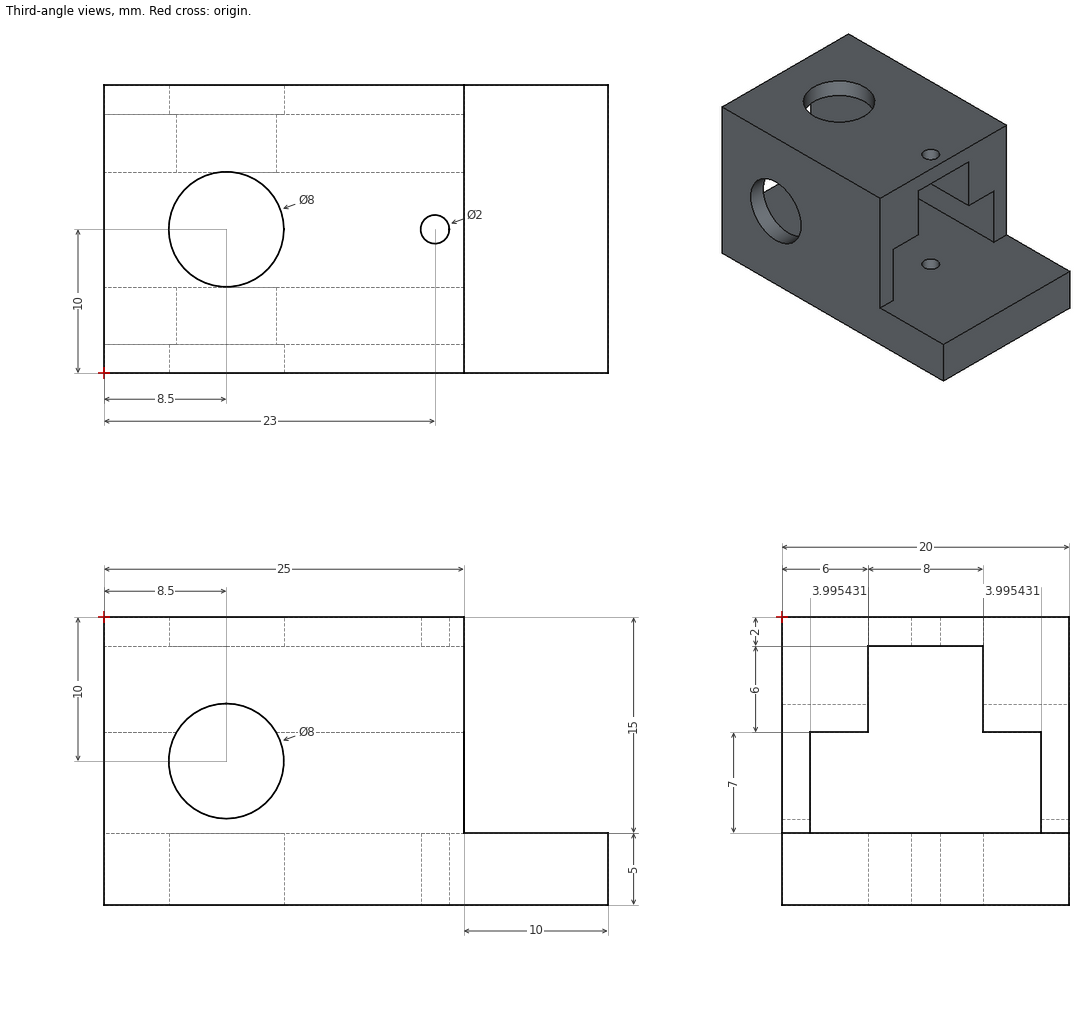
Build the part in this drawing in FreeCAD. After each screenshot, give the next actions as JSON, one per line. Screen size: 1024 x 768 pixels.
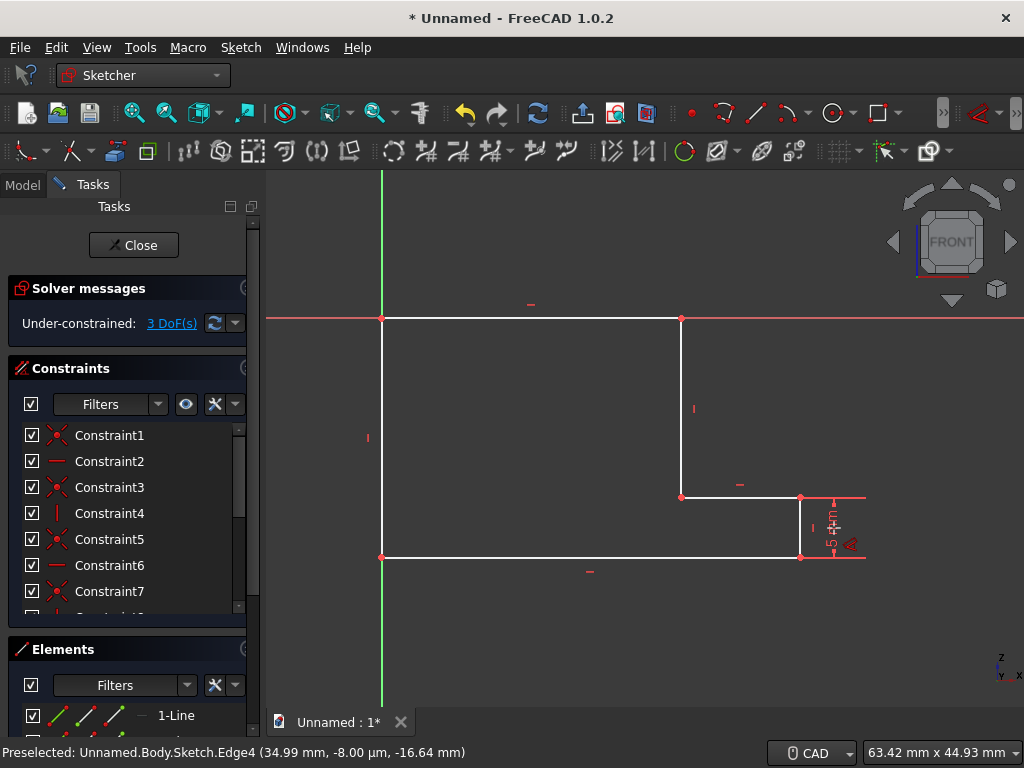
{"action": "left_click", "coordinate": [472, 318]}
{"action": "left_click", "coordinate": [531, 284]}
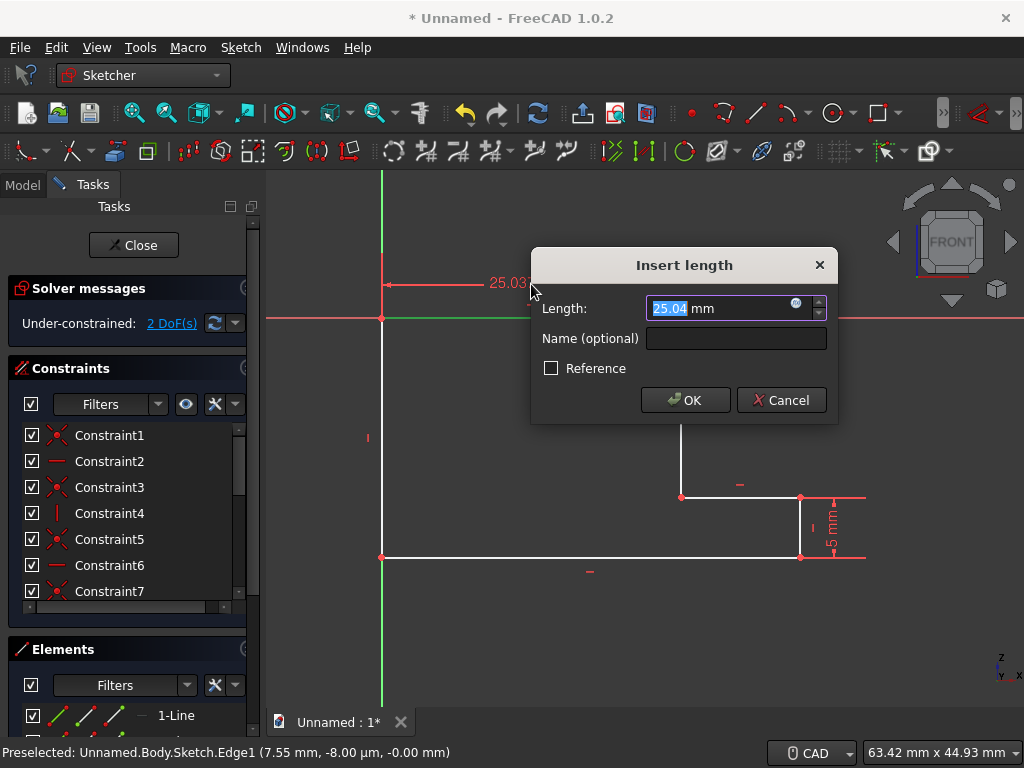
{"action": "type", "text": "25"}
{"action": "key", "text": "Return"}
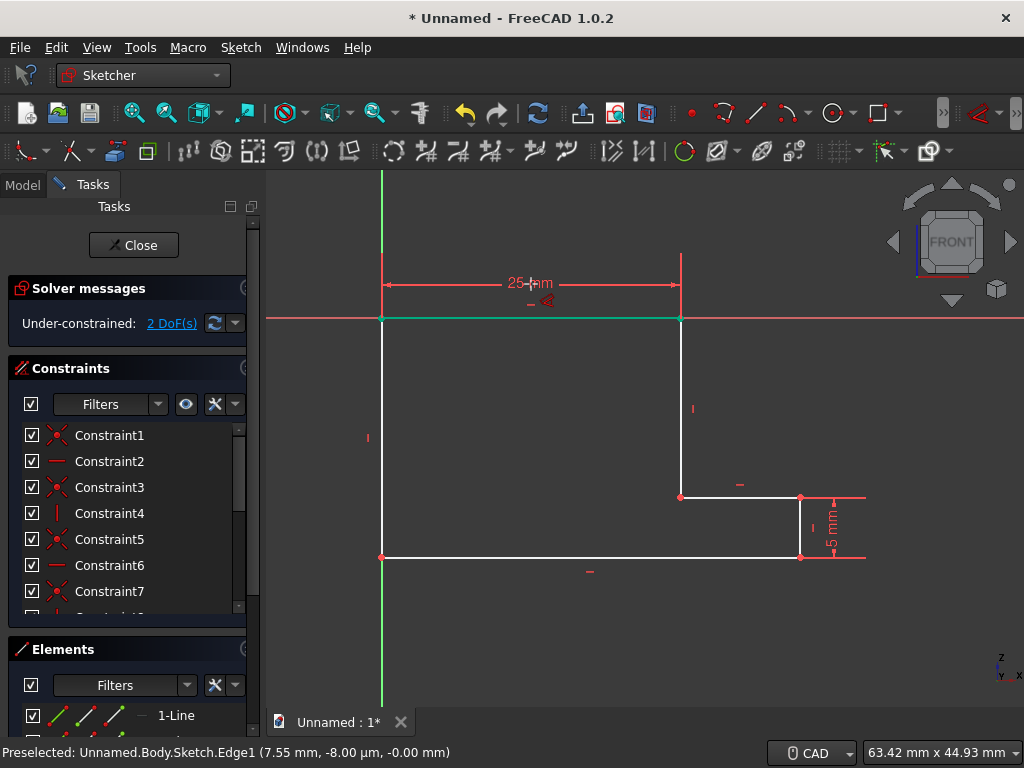
{"action": "left_click", "coordinate": [681, 372]}
{"action": "left_click", "coordinate": [715, 408]}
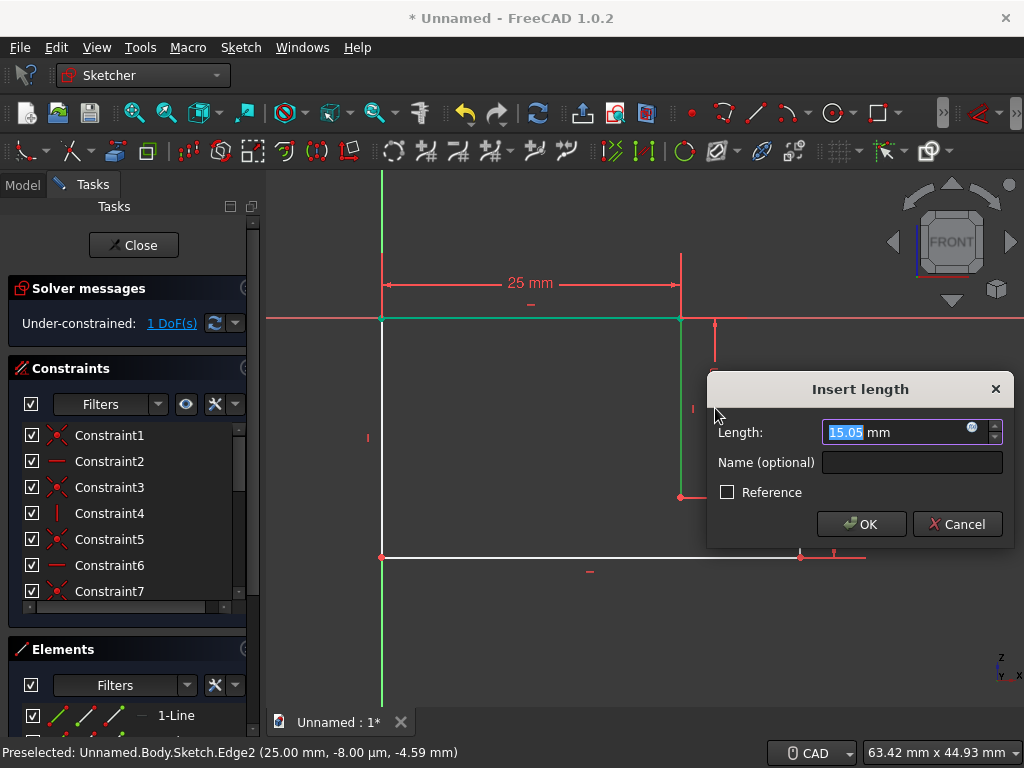
{"action": "type", "text": "15"}
{"action": "key", "text": "Return"}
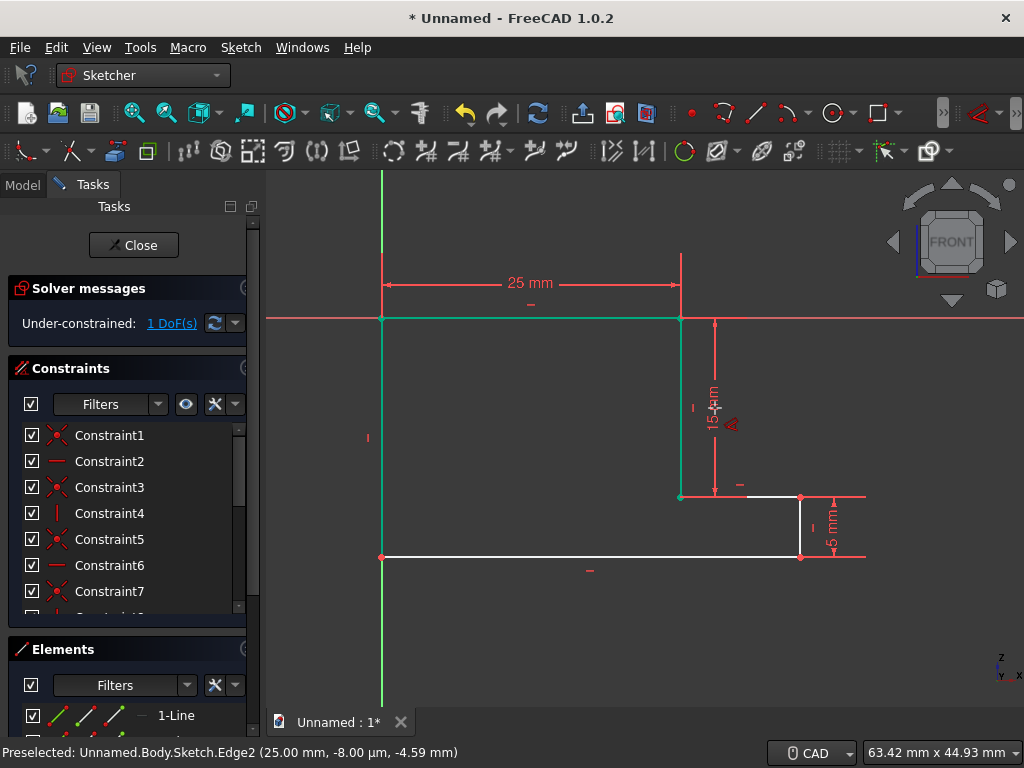
{"action": "left_click", "coordinate": [716, 497]}
{"action": "left_click", "coordinate": [740, 531]}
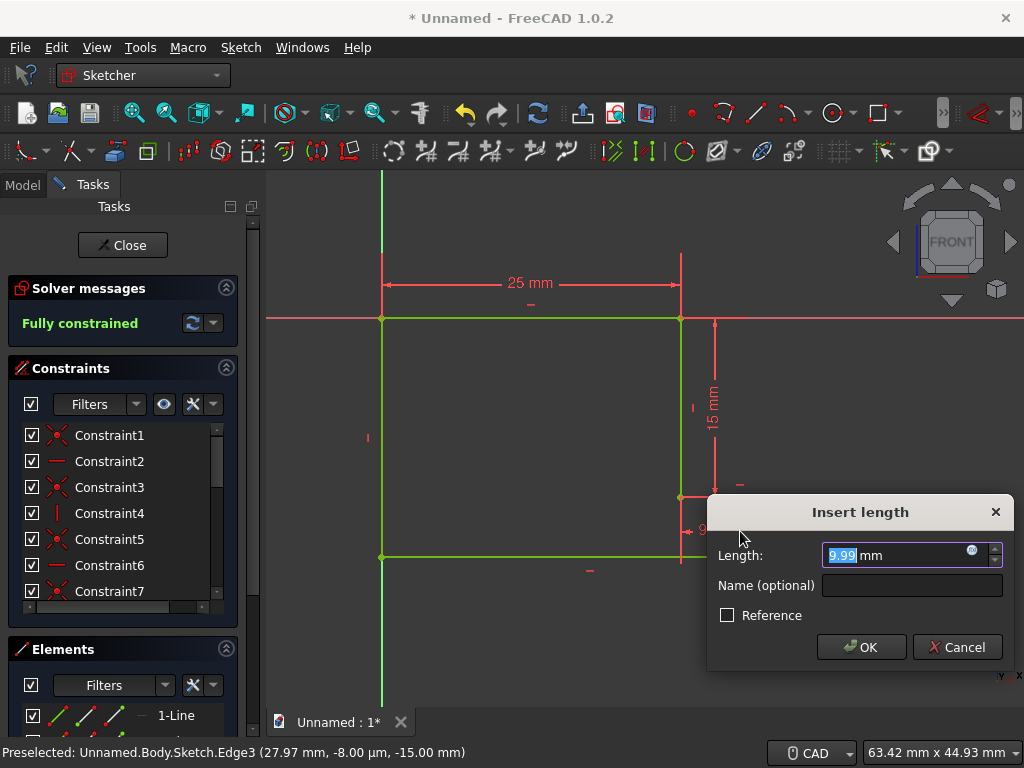
{"action": "type", "text": "10"}
{"action": "key", "text": "Return"}
{"action": "key", "text": "Escape"}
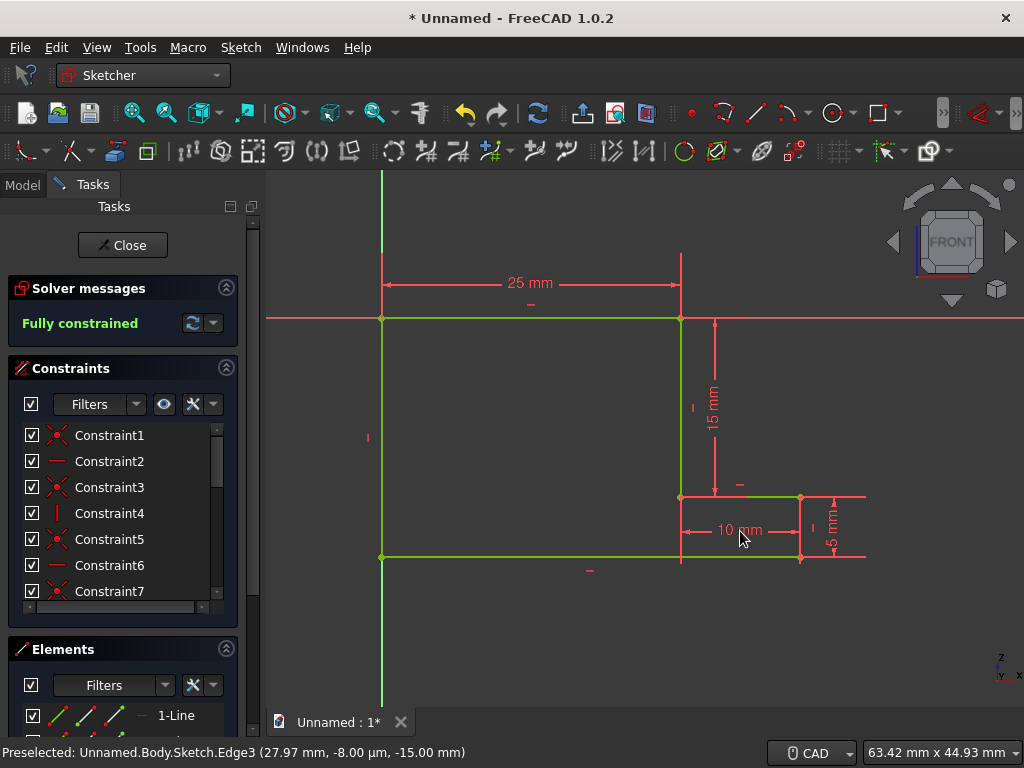
{"action": "left_click", "coordinate": [123, 245]}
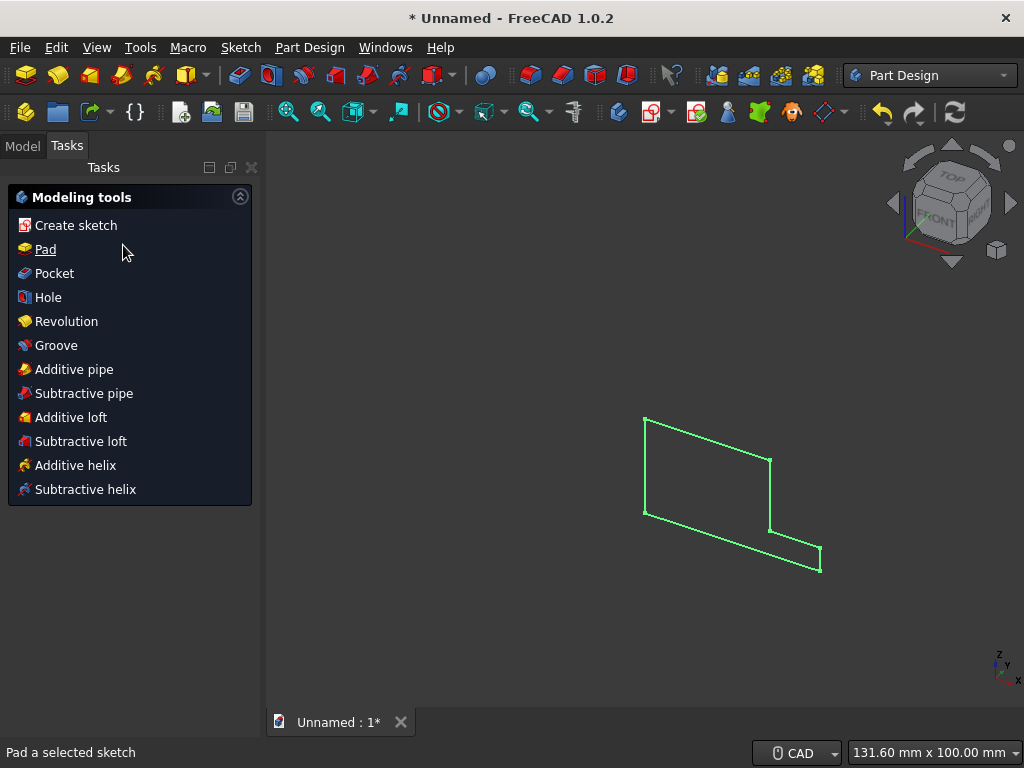
{"action": "left_click", "coordinate": [26, 76]}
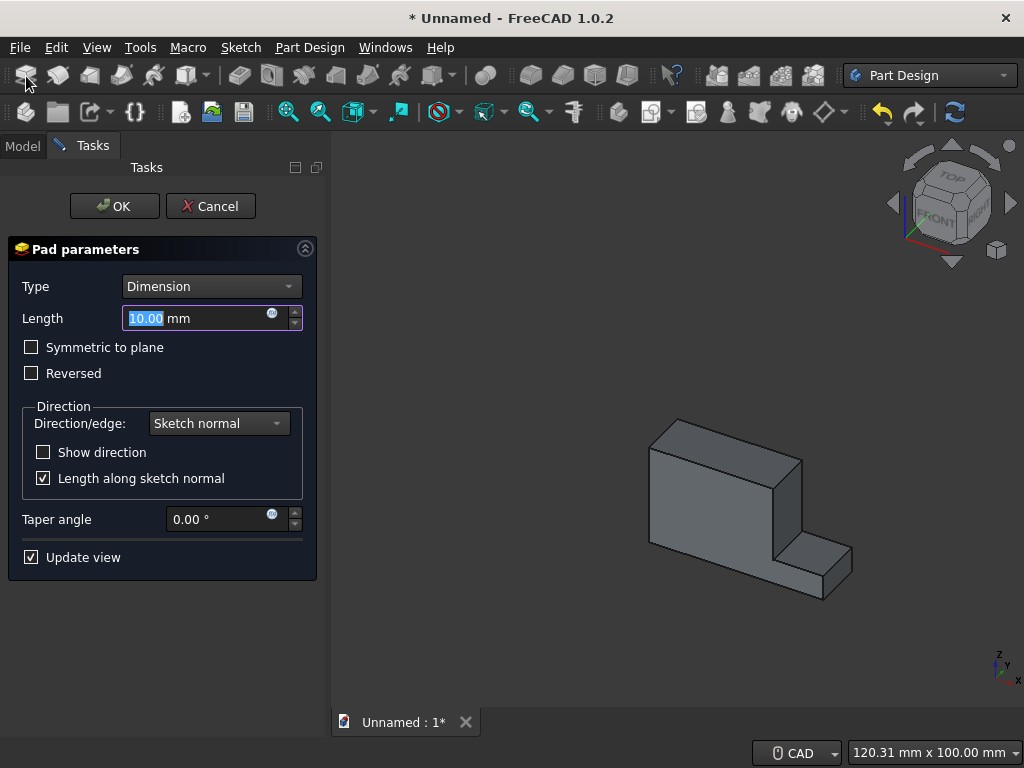
{"action": "type", "text": "20"}
{"action": "key", "text": "Tab"}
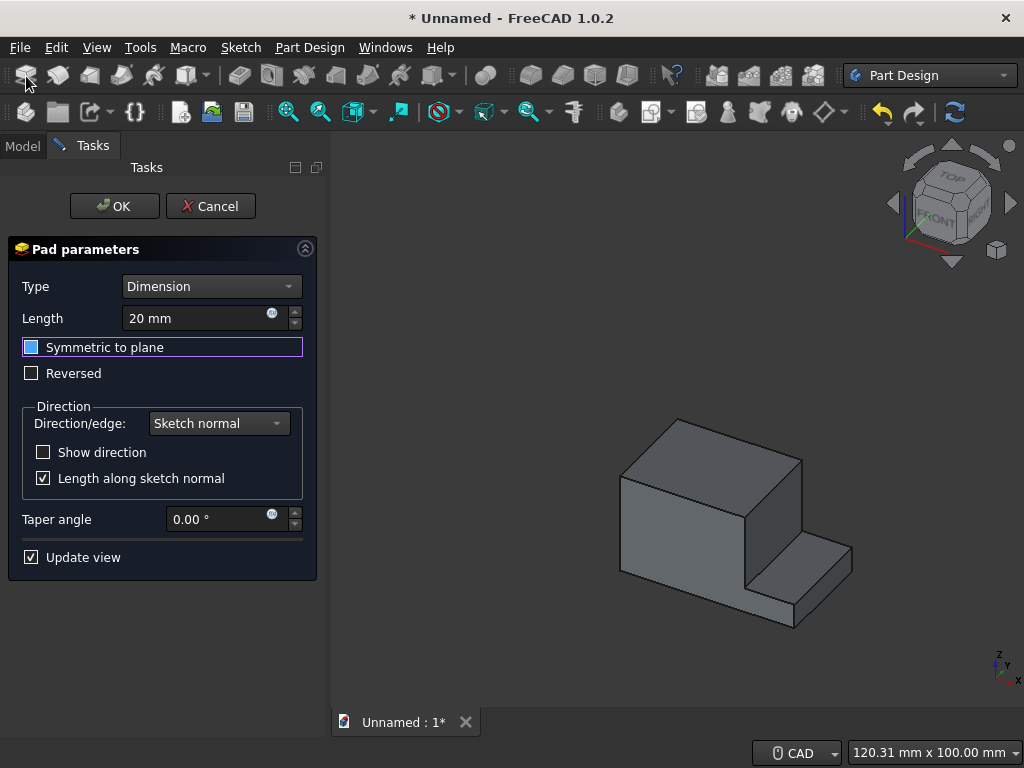
{"action": "left_click", "coordinate": [30, 373]}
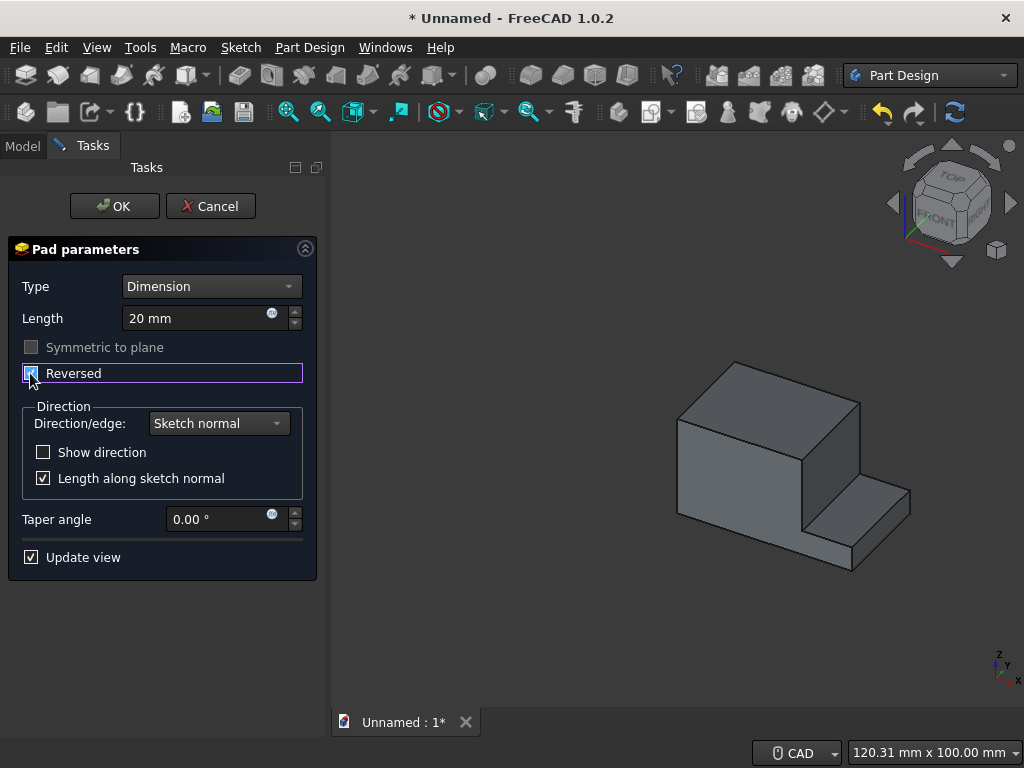
{"action": "left_click", "coordinate": [115, 206]}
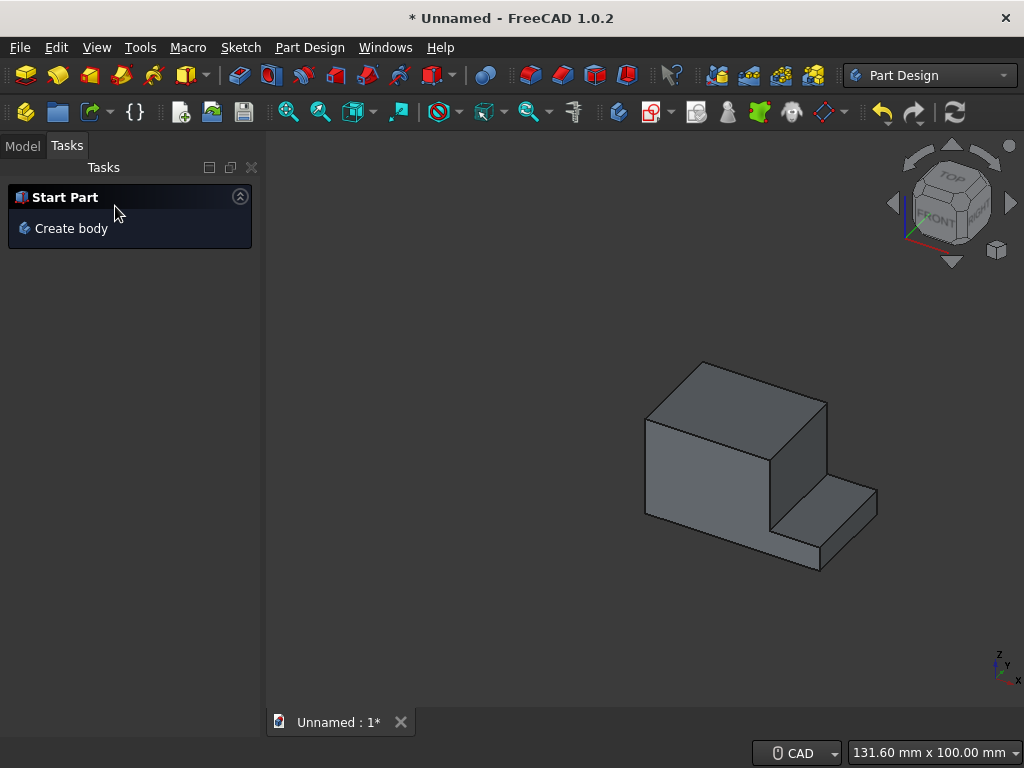
{"action": "left_click", "coordinate": [290, 112]}